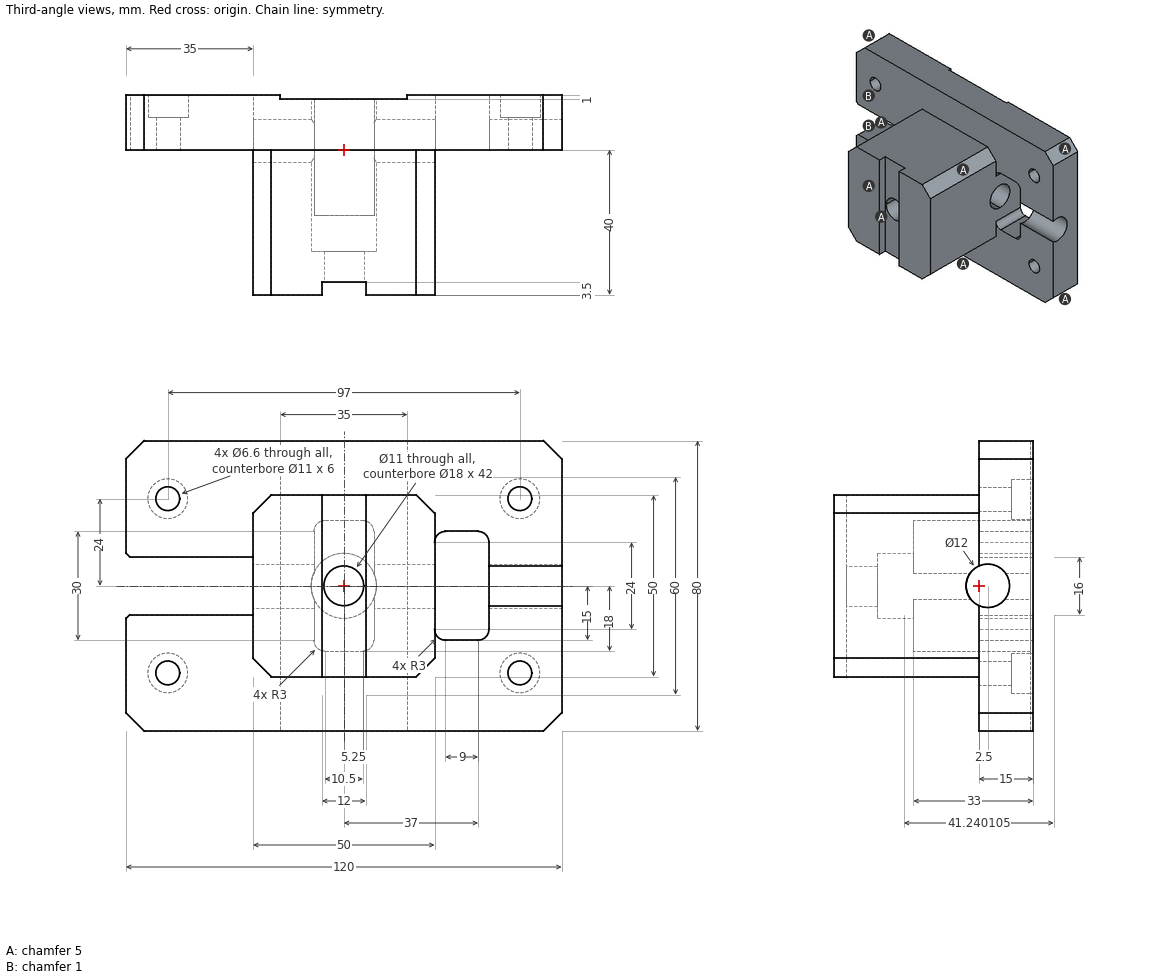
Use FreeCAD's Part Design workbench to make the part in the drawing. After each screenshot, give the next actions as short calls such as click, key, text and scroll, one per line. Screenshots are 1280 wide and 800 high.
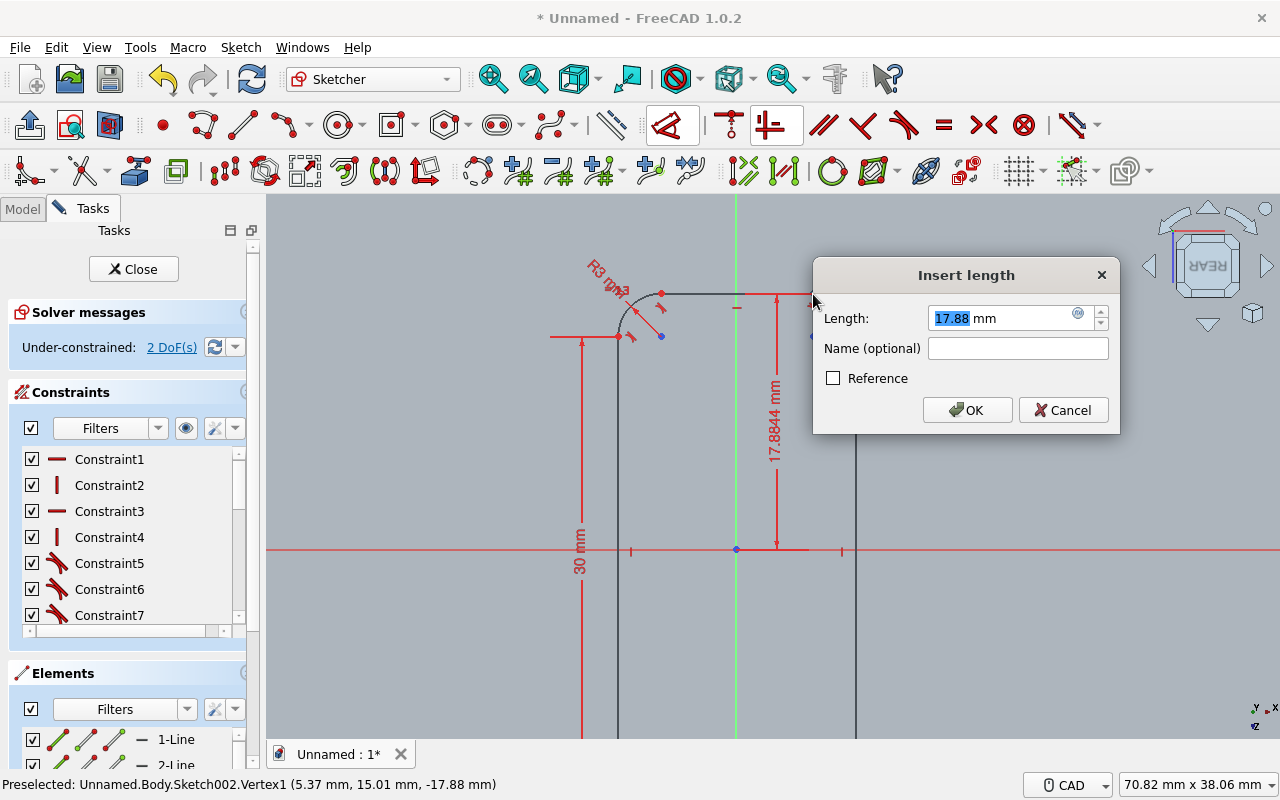
text(18)
key(Return)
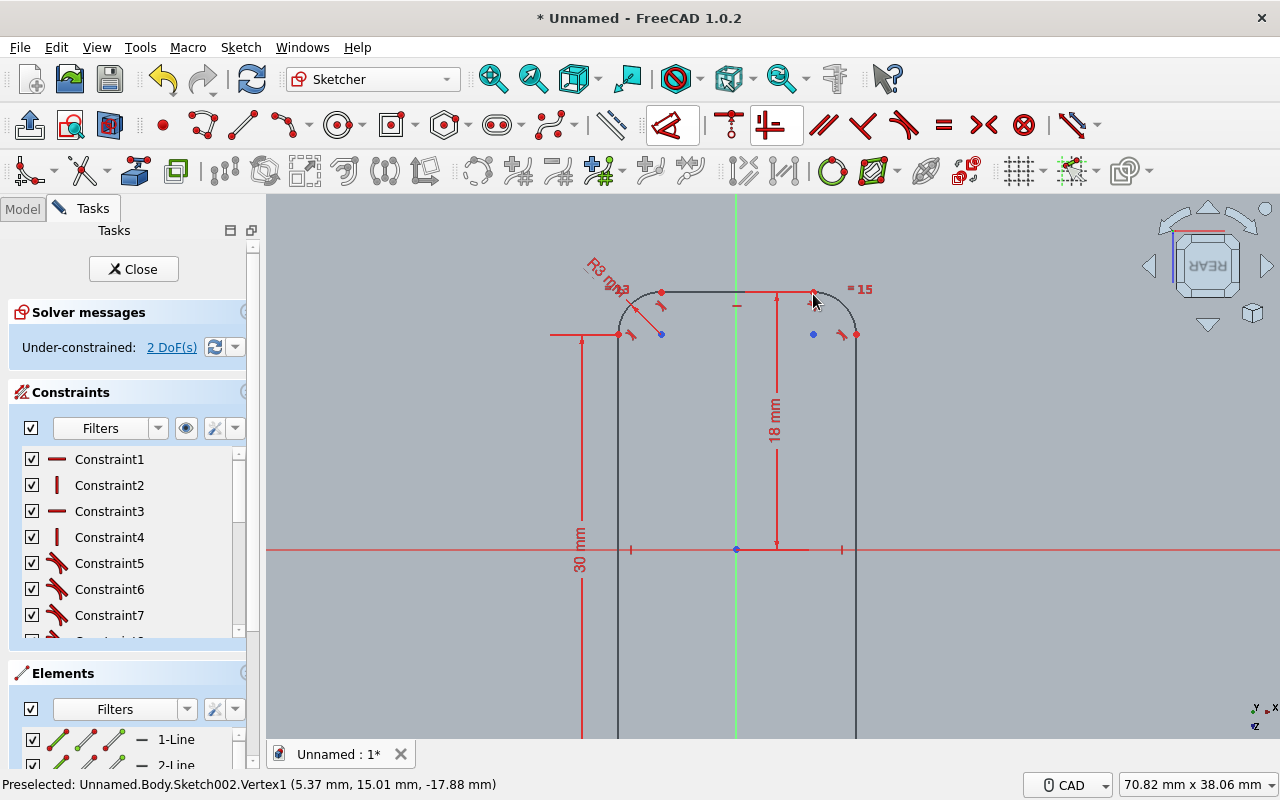
click(768, 292)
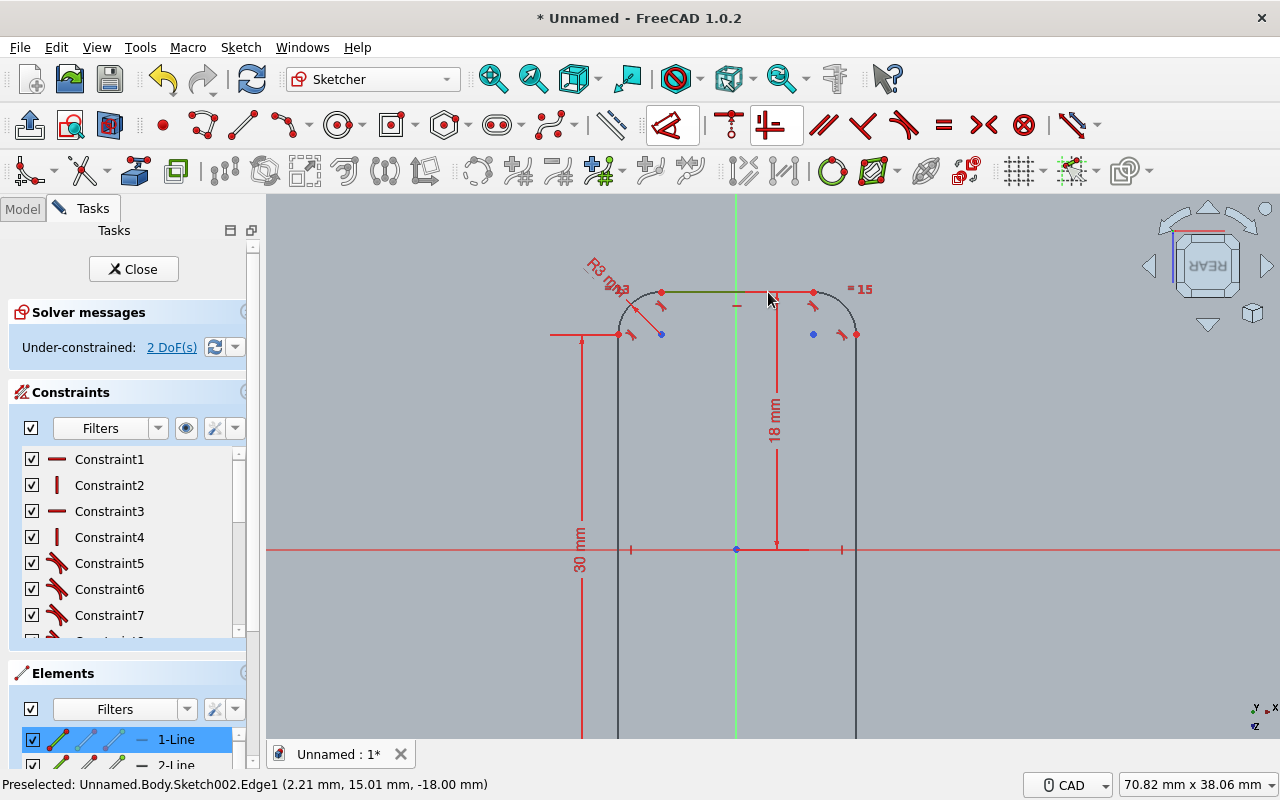
key(l)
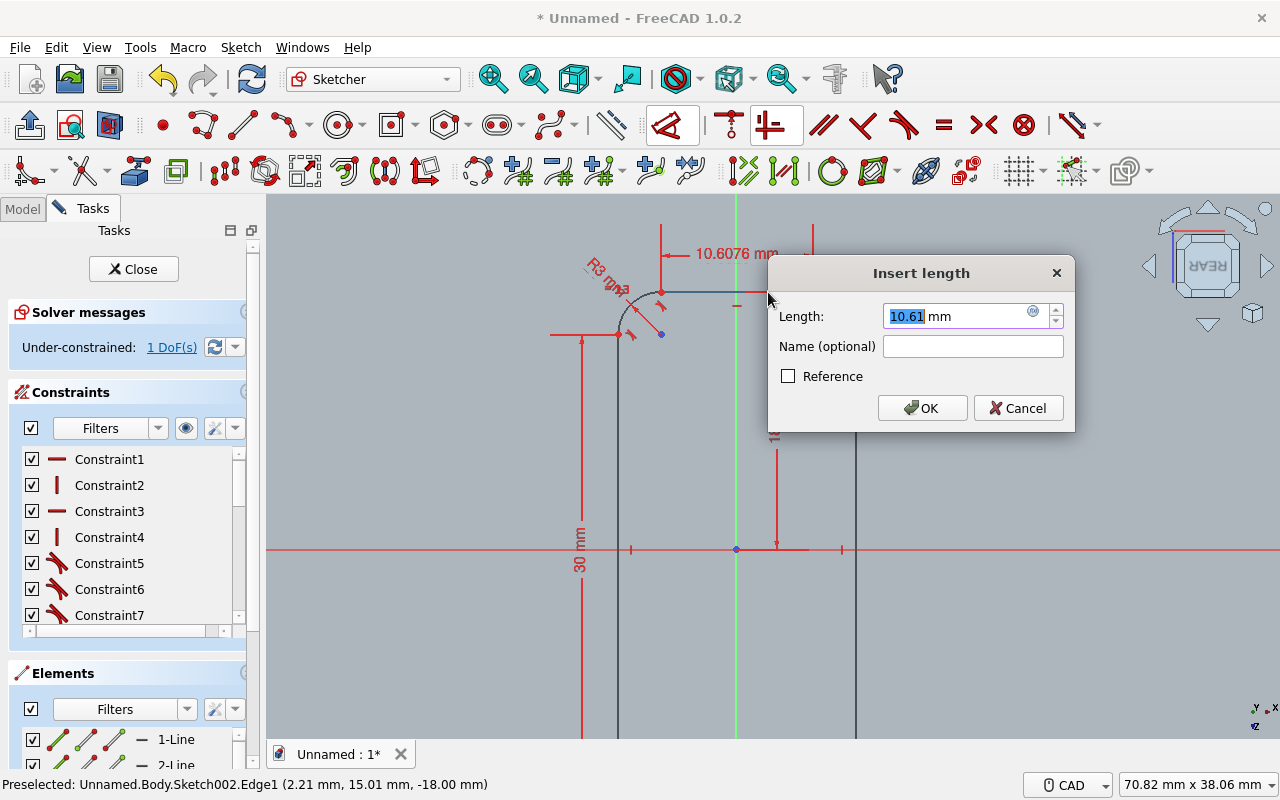
text(10.5)
key(Return)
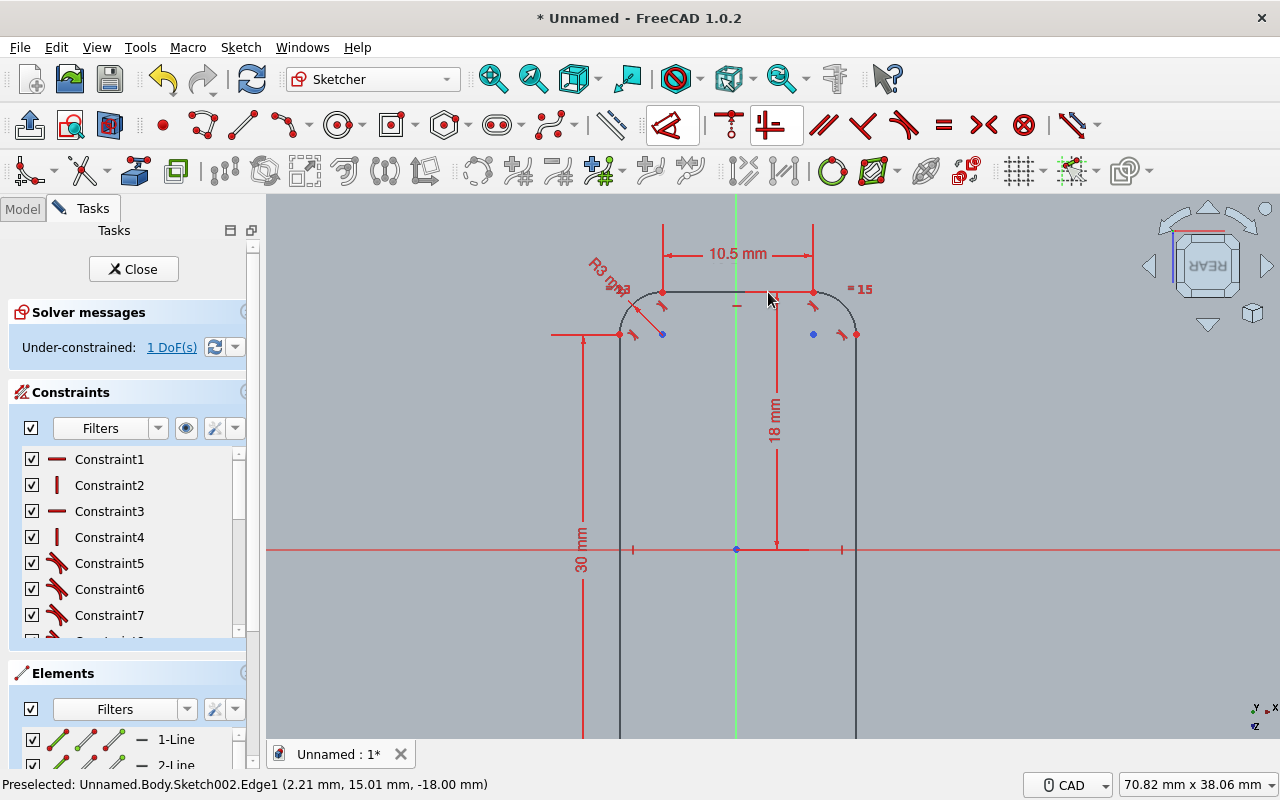
click(813, 292)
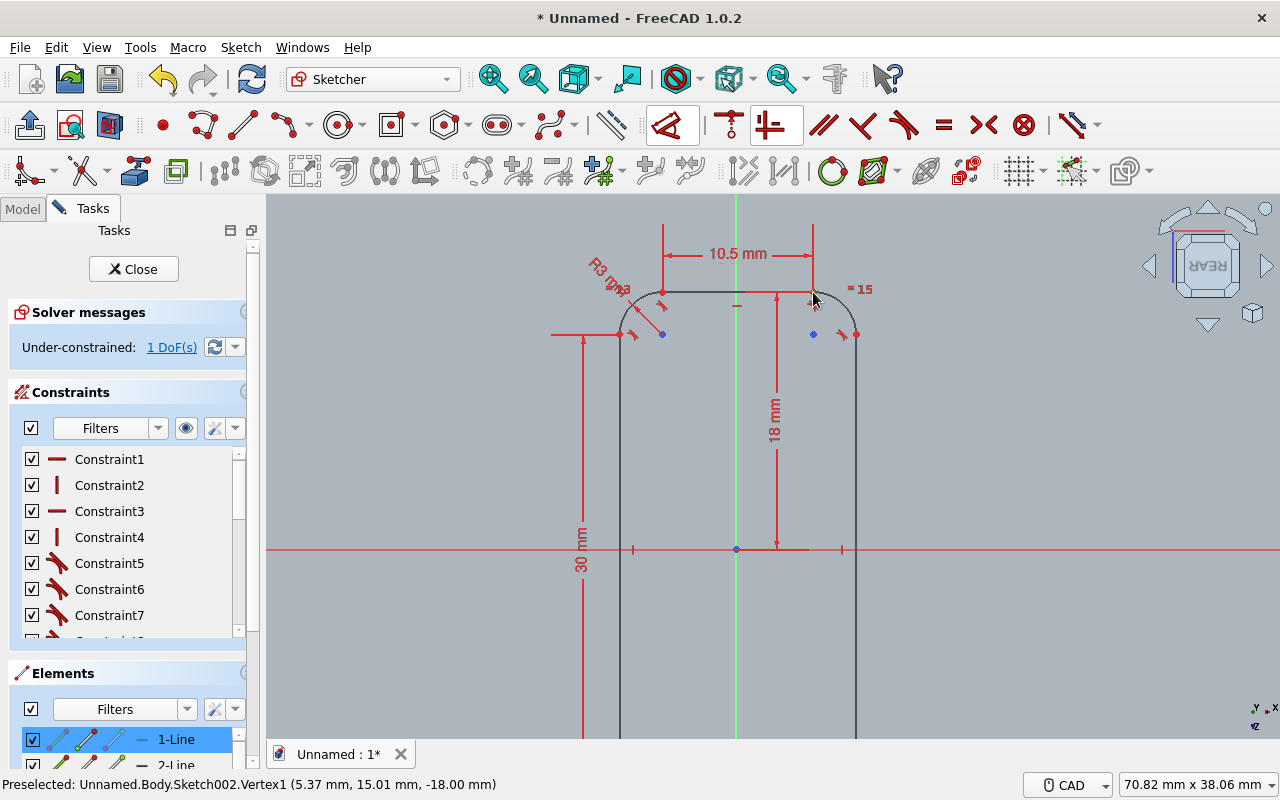
key(l)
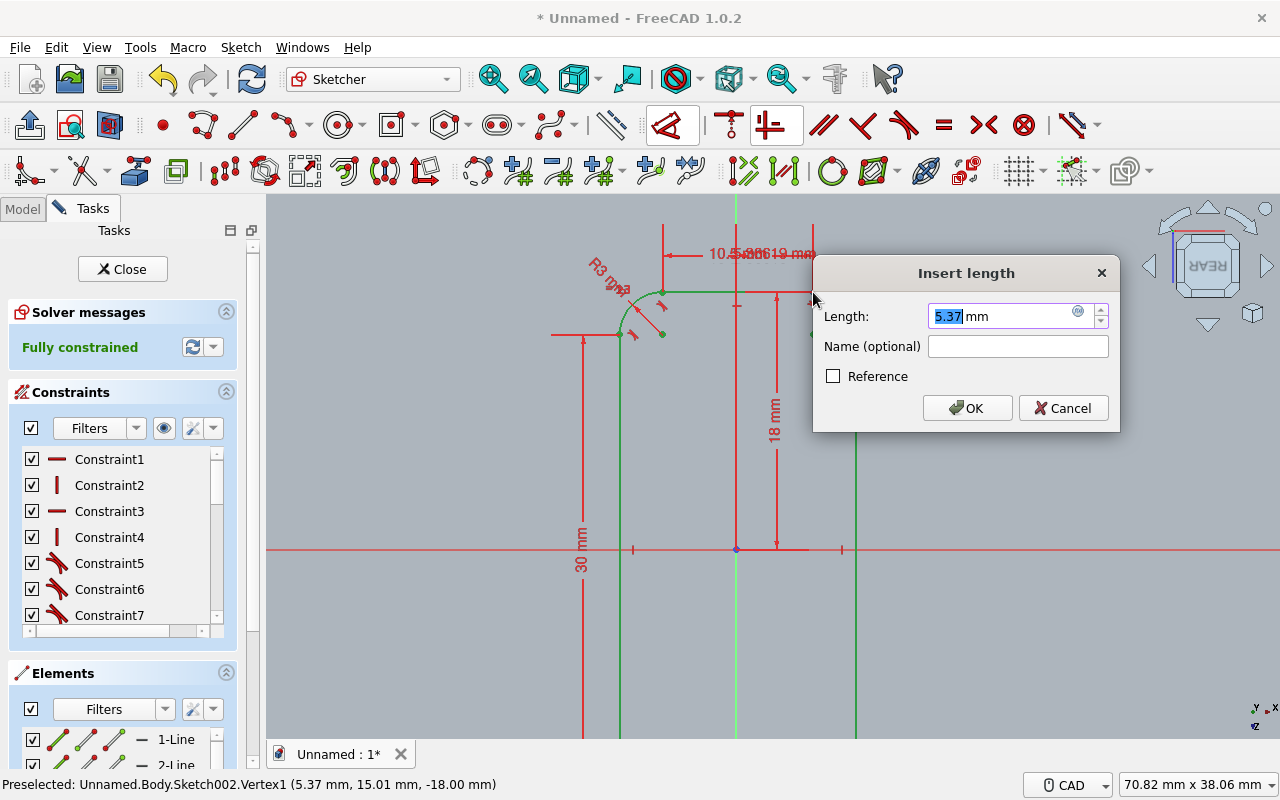
text(5.25)
key(Return)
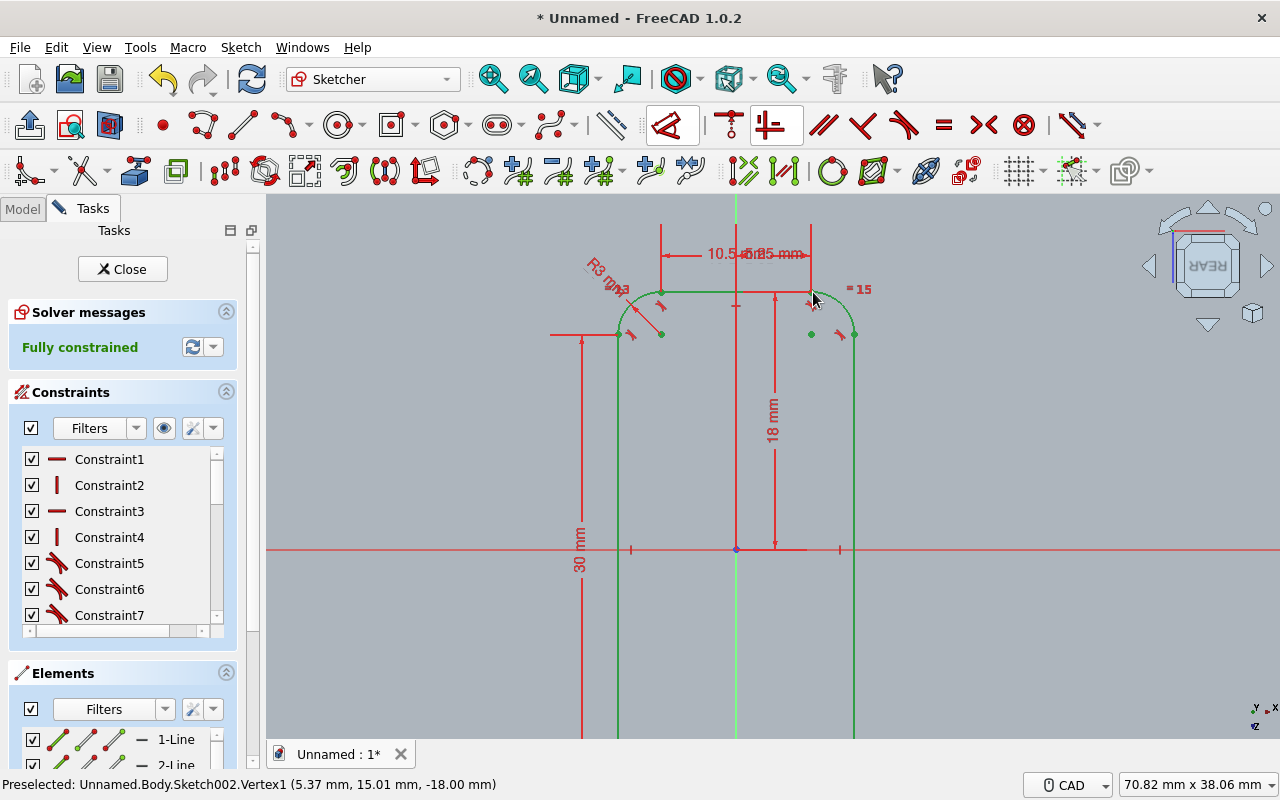
click(123, 269)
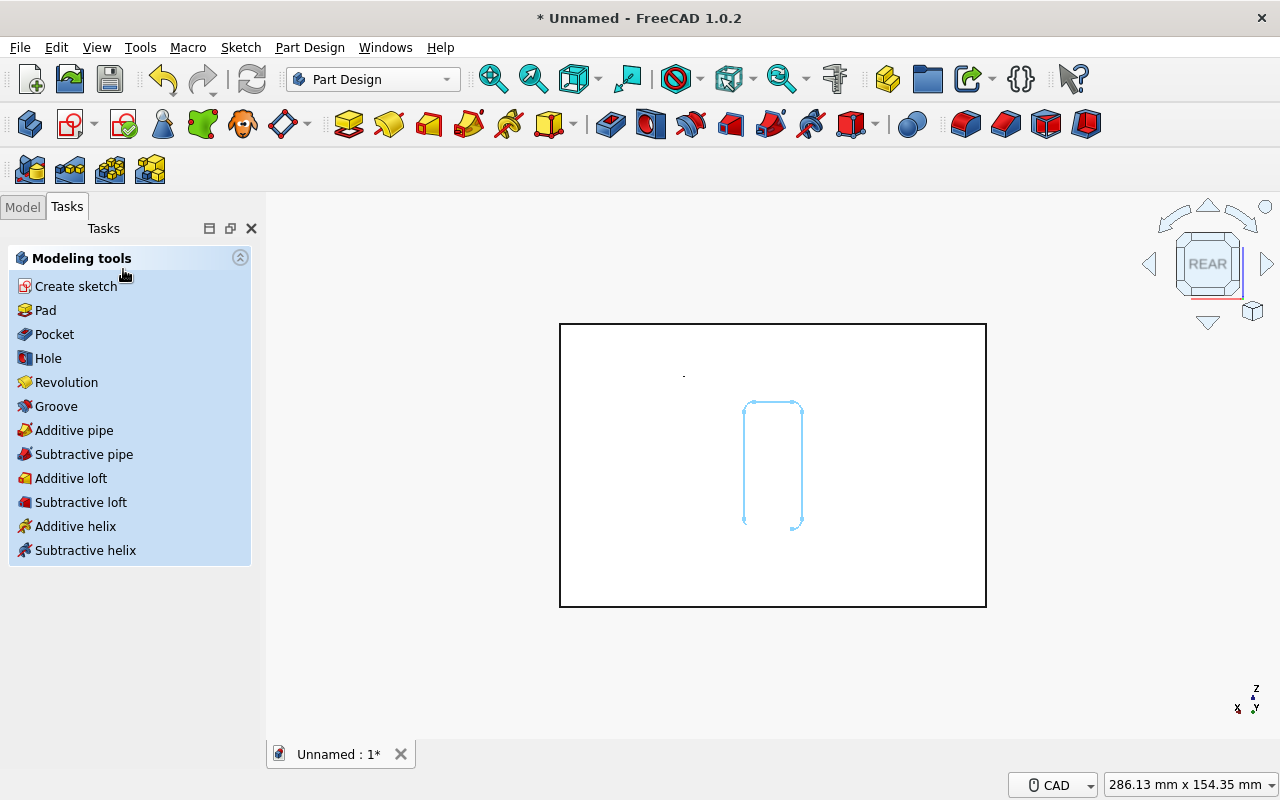
click(612, 124)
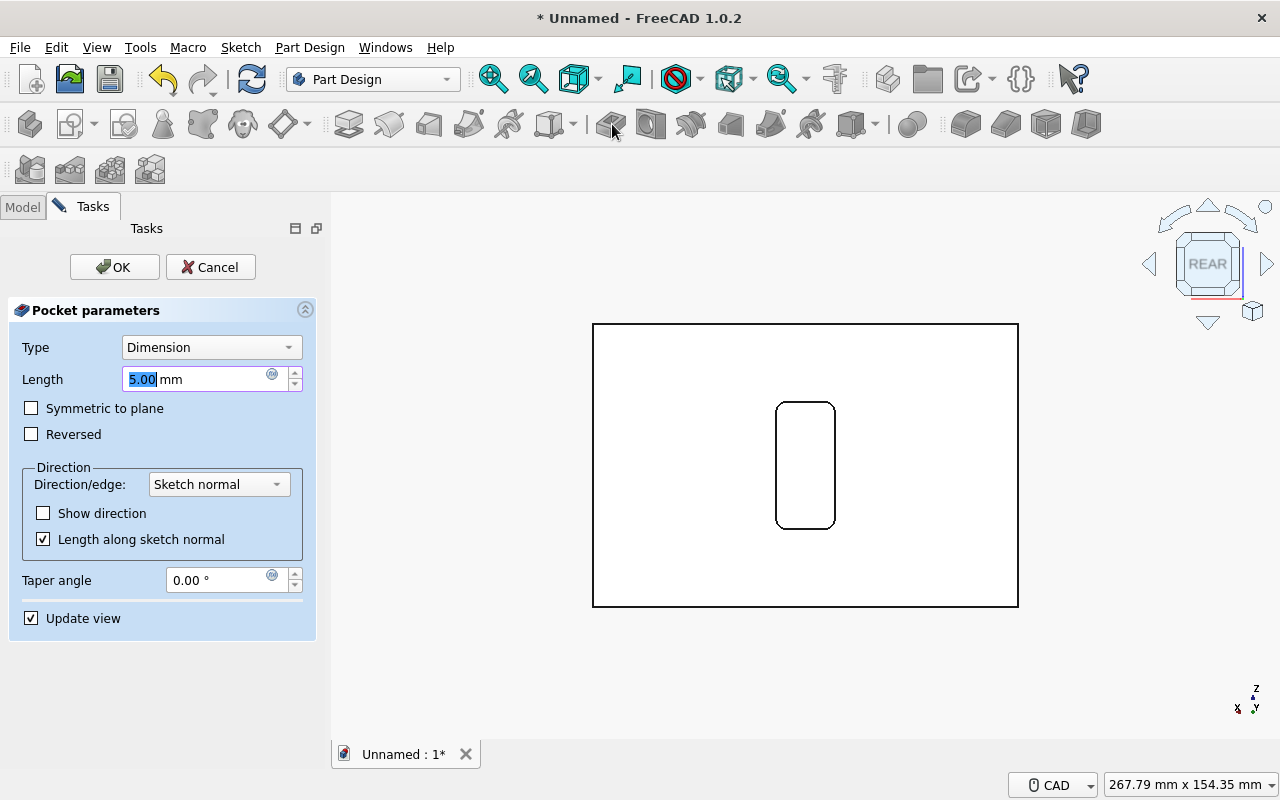
text(33)
key(Tab)